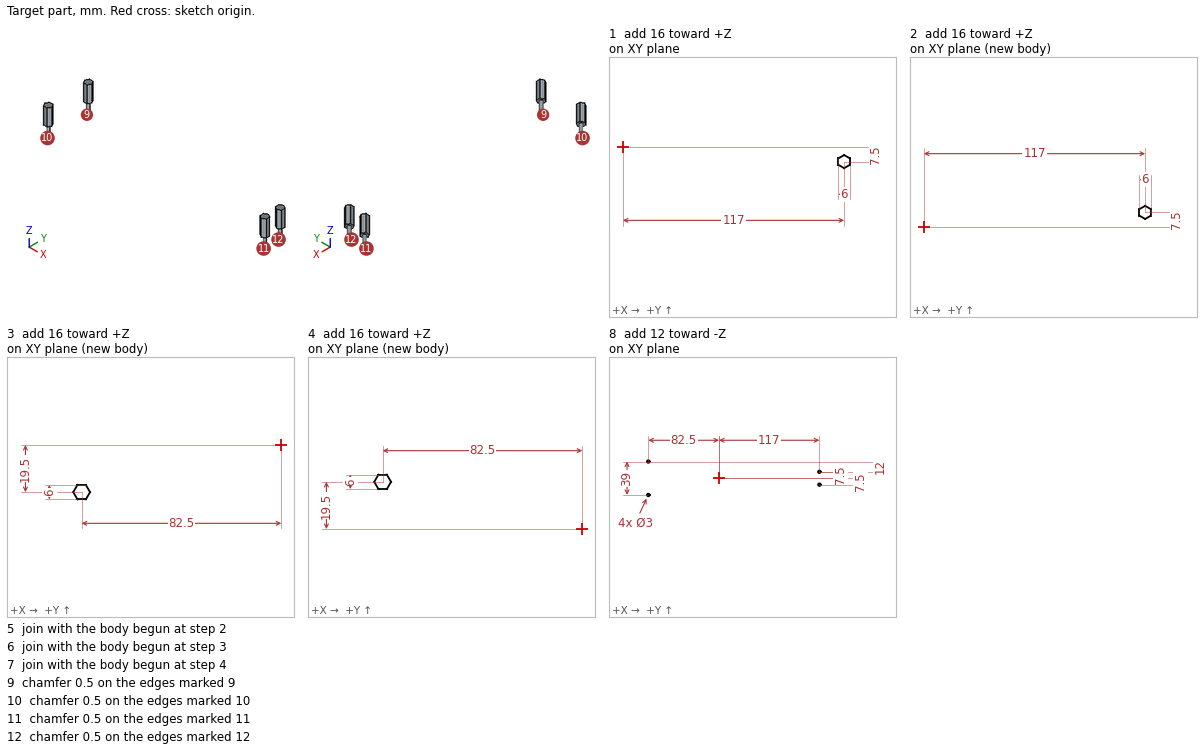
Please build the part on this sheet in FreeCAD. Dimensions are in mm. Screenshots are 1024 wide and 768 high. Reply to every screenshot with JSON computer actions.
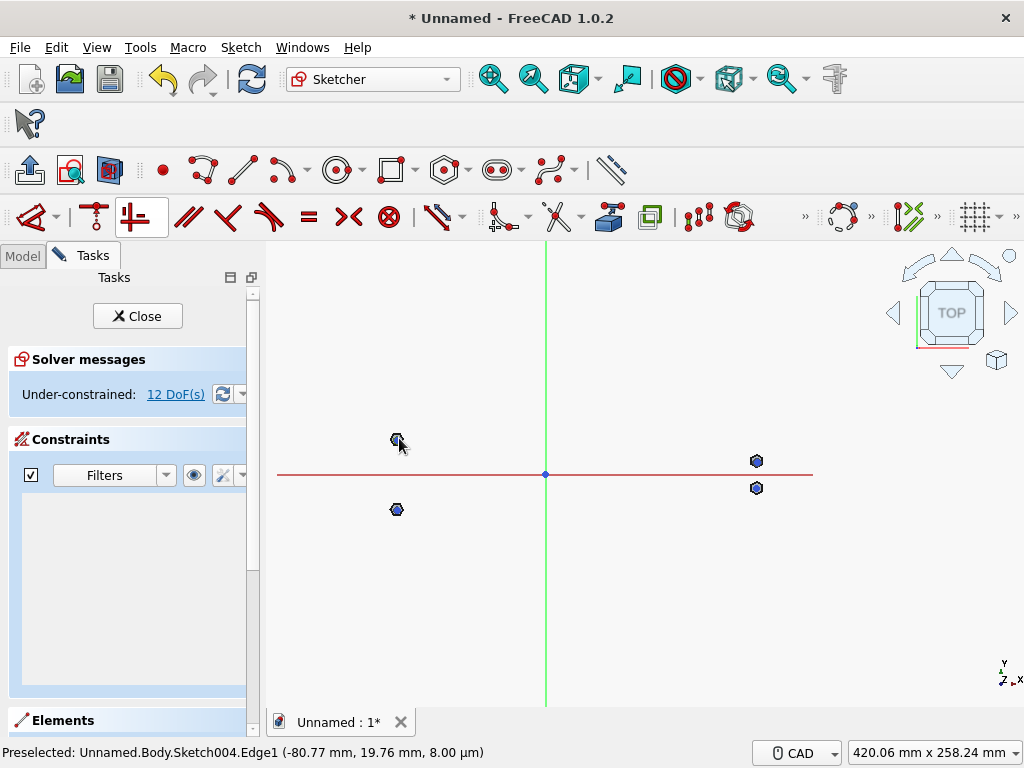
{"action": "scroll", "coordinate": [399, 508], "scroll_direction": "up", "scroll_amount": 8}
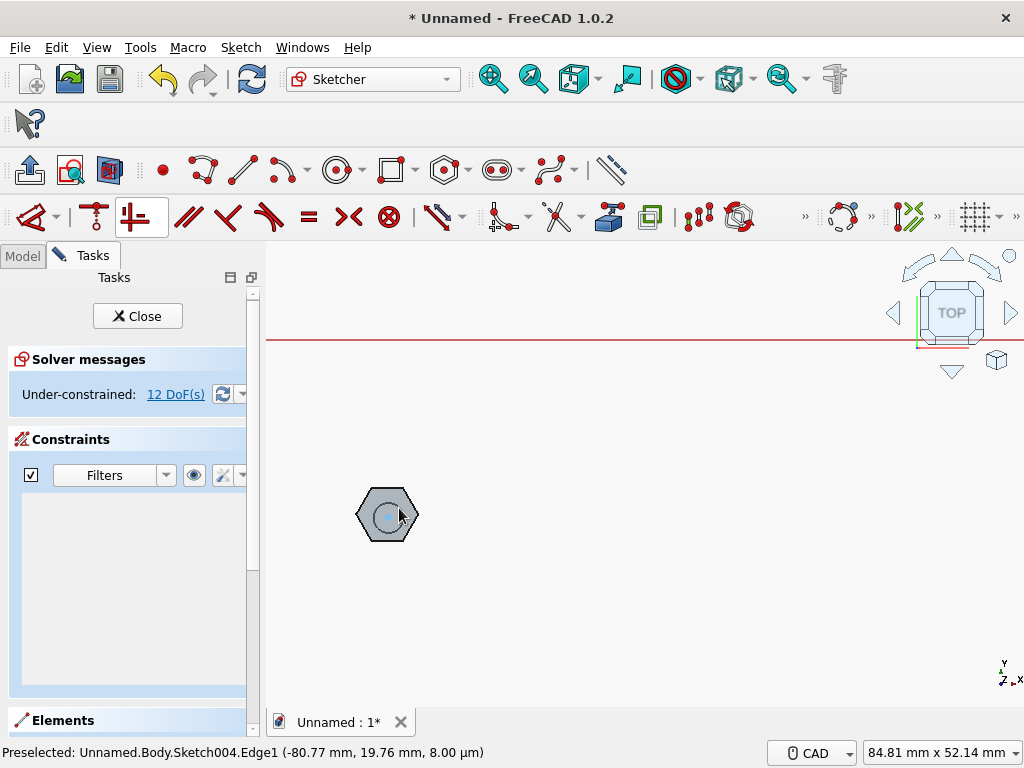
{"action": "left_click", "coordinate": [399, 507]}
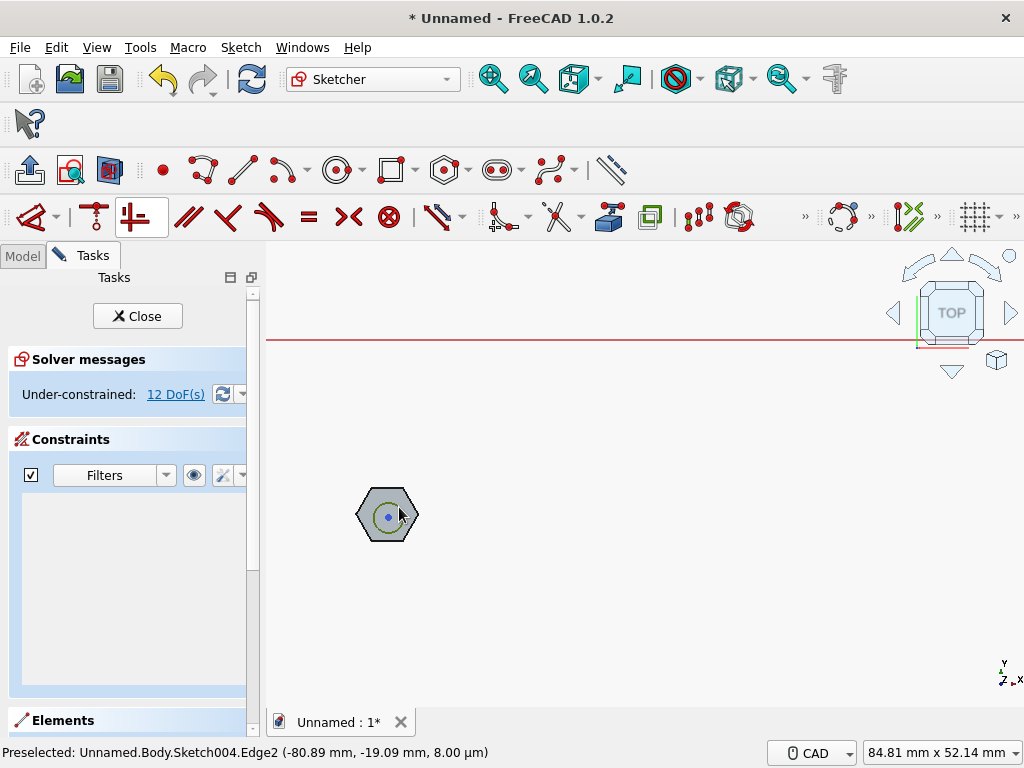
{"action": "scroll", "coordinate": [399, 508], "scroll_direction": "down", "scroll_amount": 8}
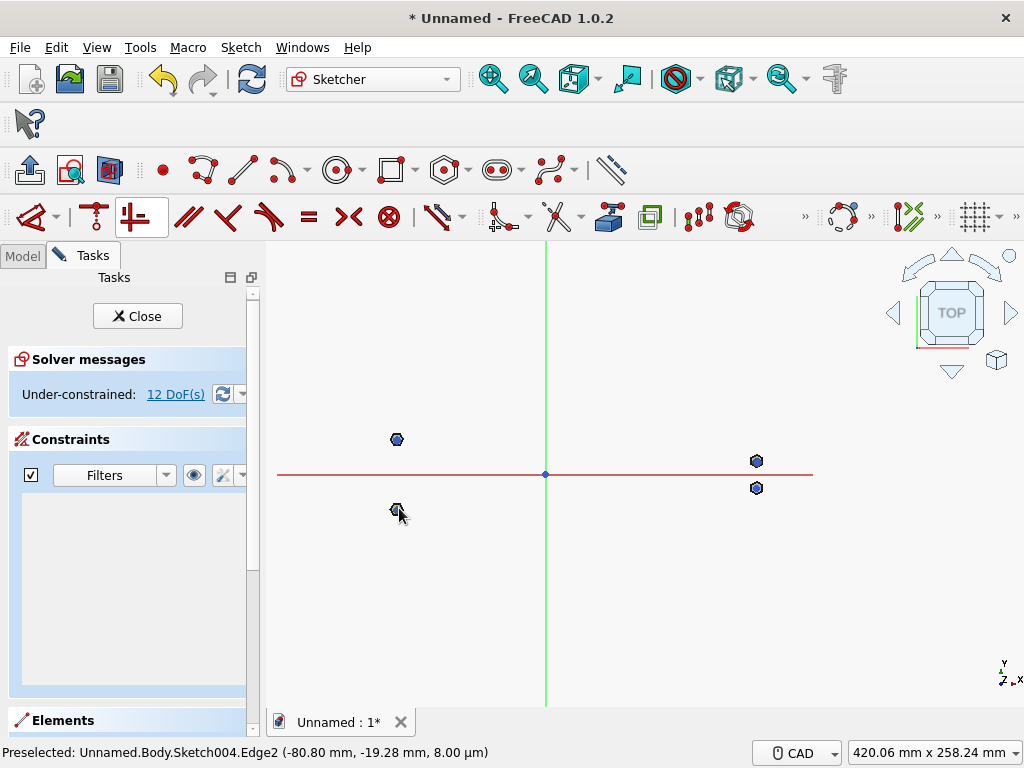
{"action": "scroll", "coordinate": [760, 460], "scroll_direction": "up", "scroll_amount": 7}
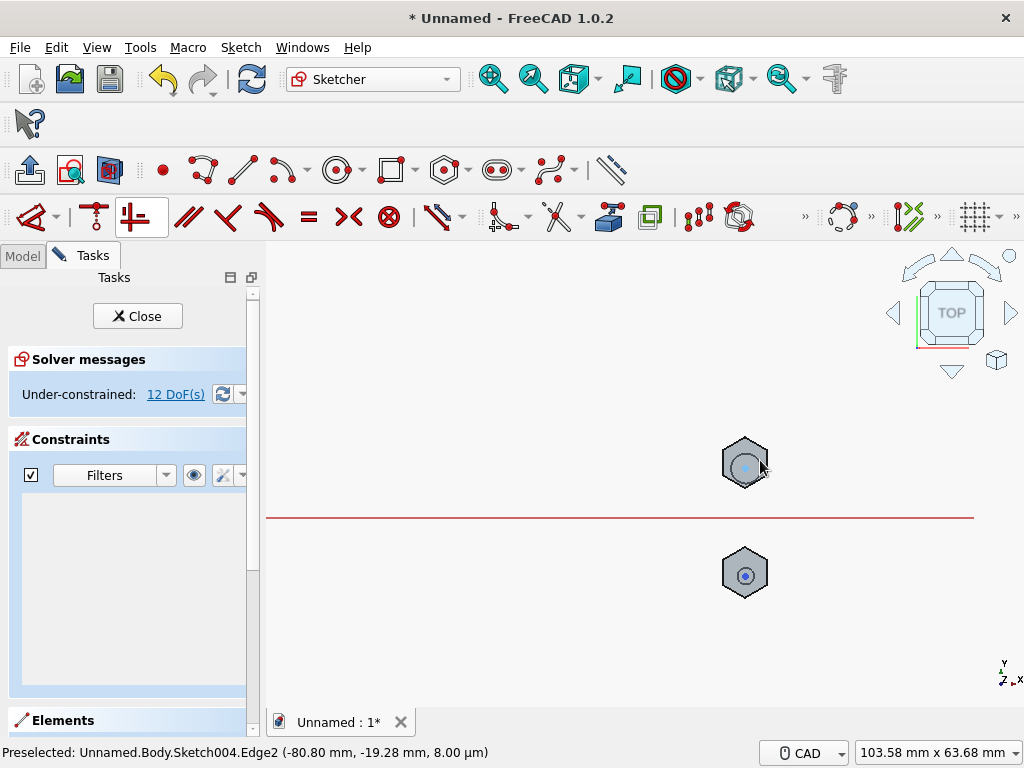
{"action": "left_click", "coordinate": [757, 458]}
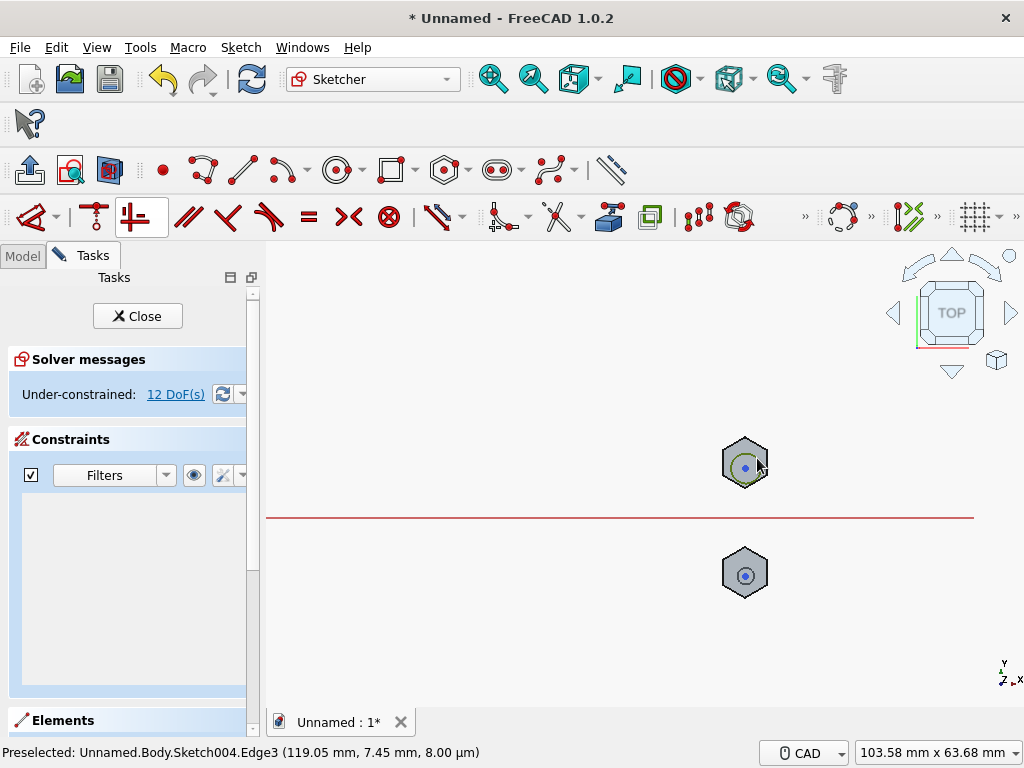
{"action": "scroll", "coordinate": [752, 570], "scroll_direction": "up", "scroll_amount": 3}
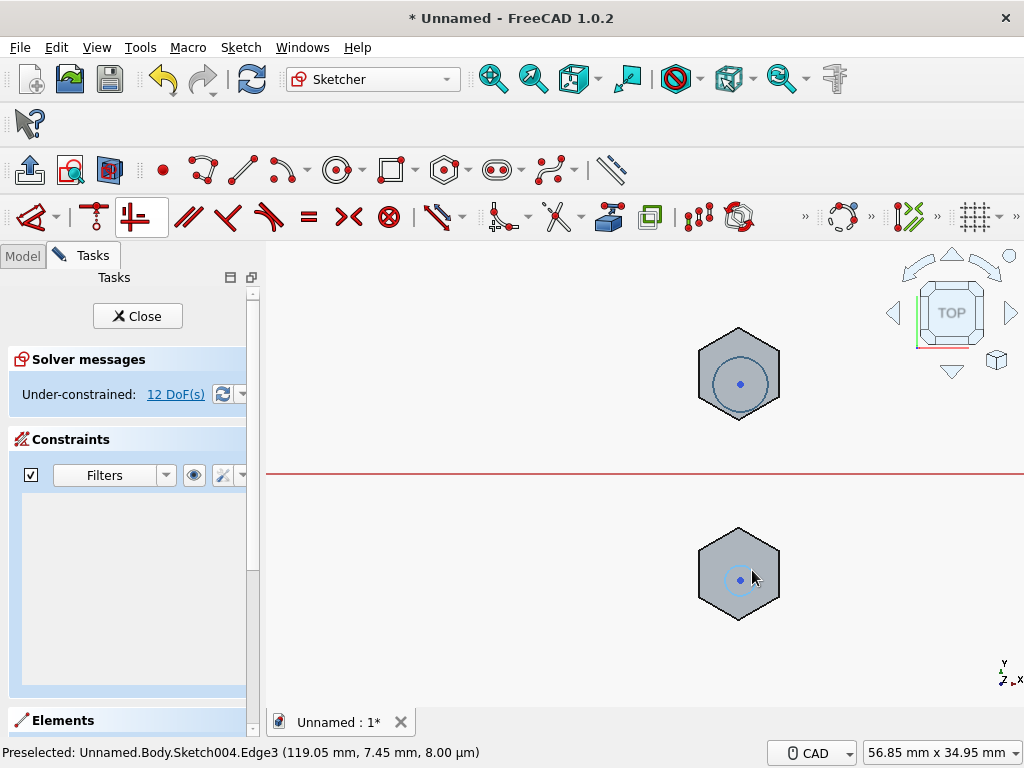
{"action": "left_click", "coordinate": [751, 570]}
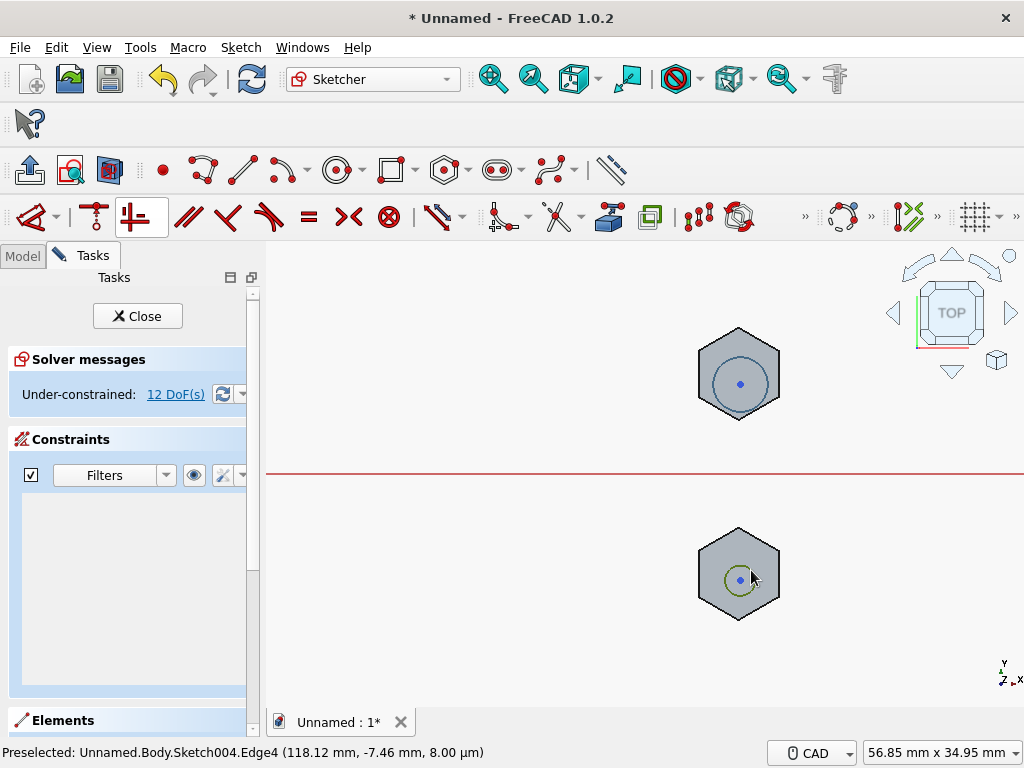
{"action": "left_click", "coordinate": [310, 218]}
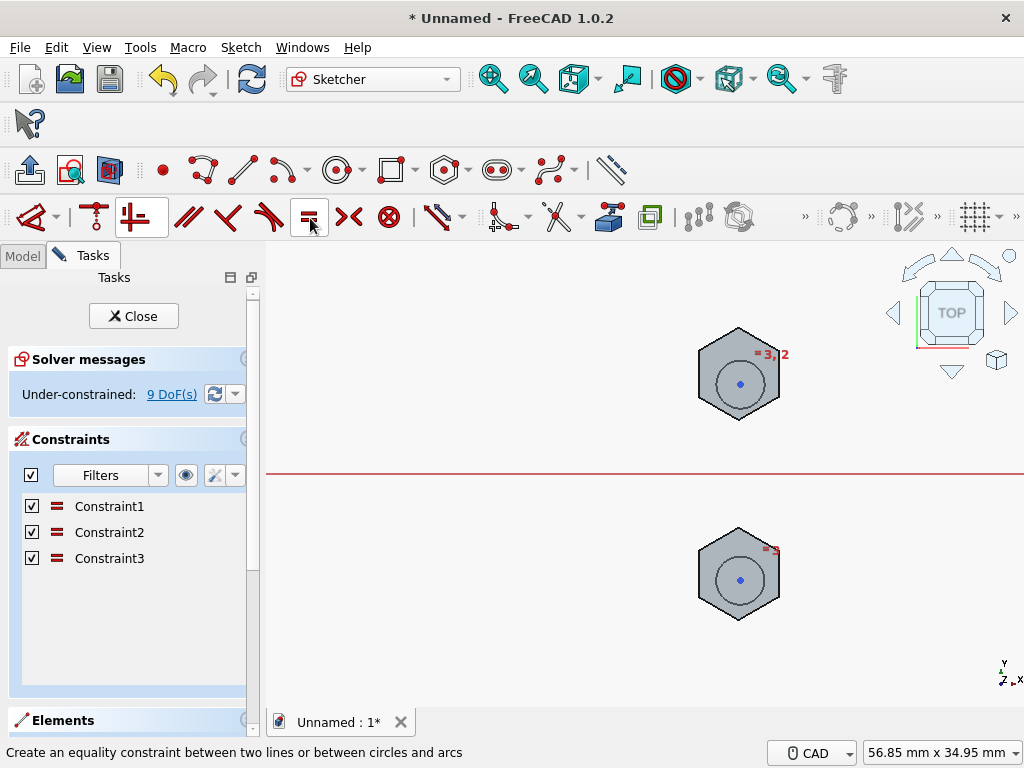
{"action": "scroll", "coordinate": [759, 474], "scroll_direction": "down", "scroll_amount": 10}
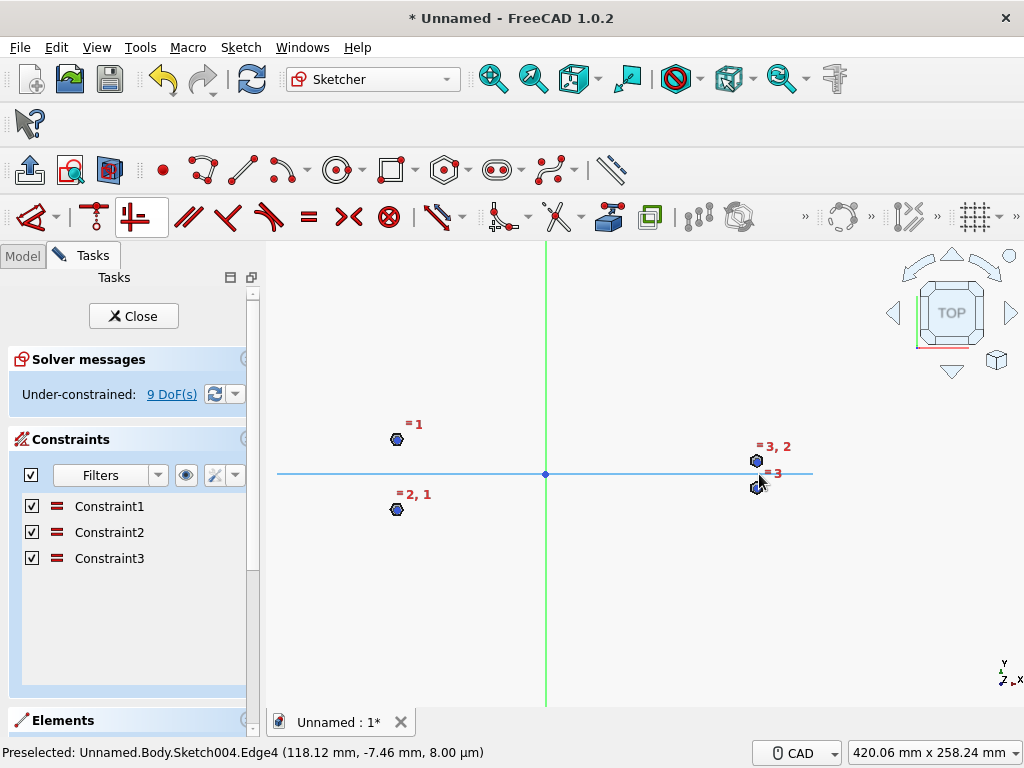
{"action": "left_click", "coordinate": [397, 440]}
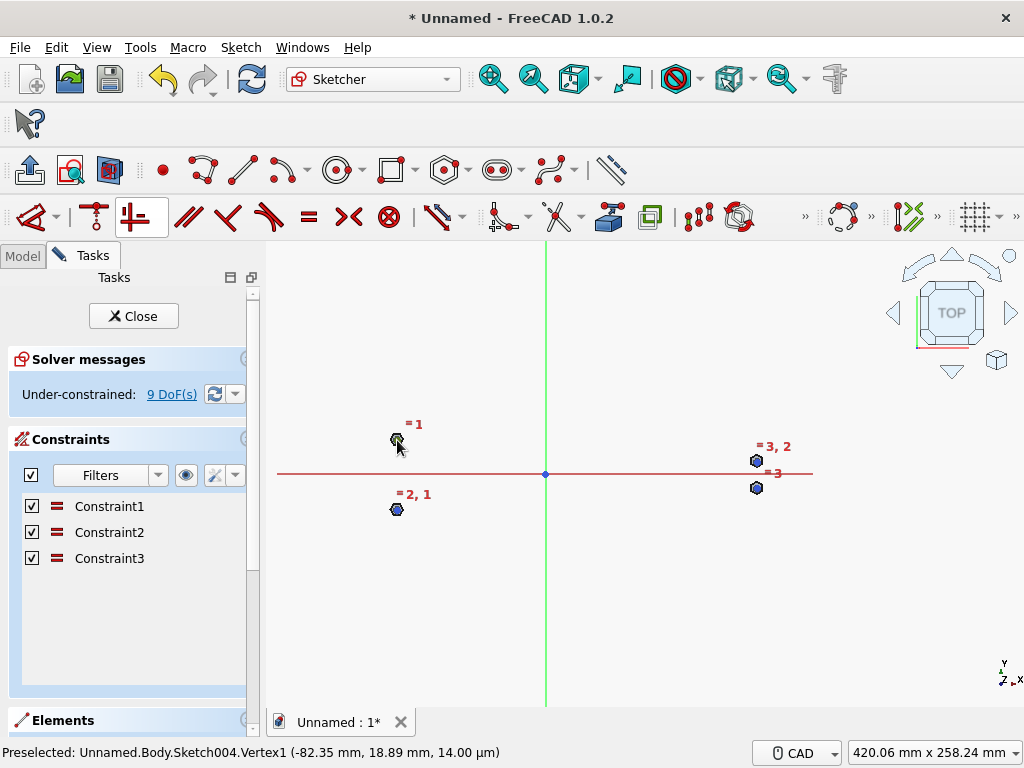
{"action": "left_click", "coordinate": [397, 510]}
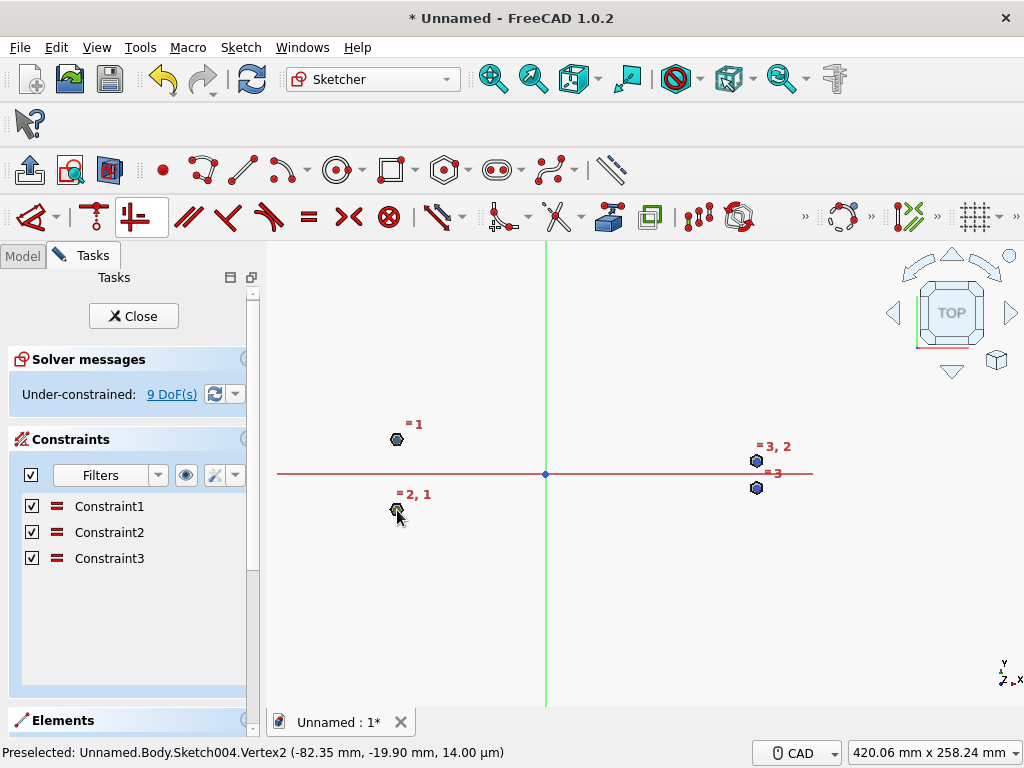
{"action": "left_click", "coordinate": [162, 218]}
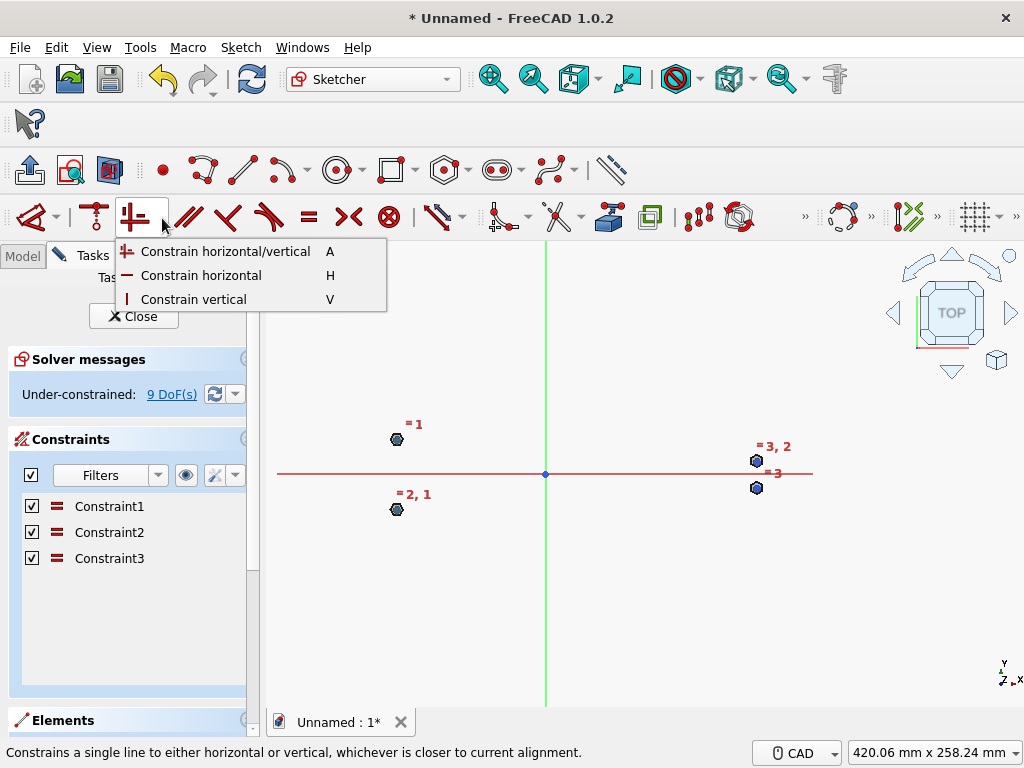
{"action": "left_click", "coordinate": [251, 299]}